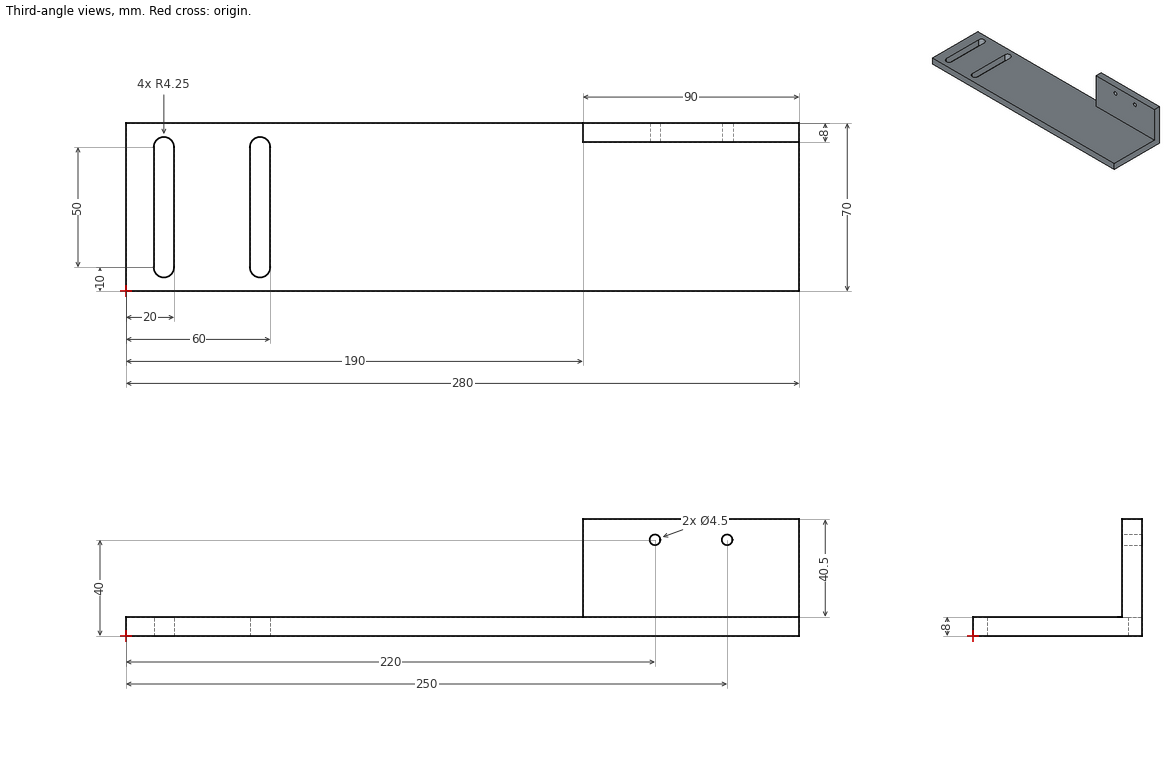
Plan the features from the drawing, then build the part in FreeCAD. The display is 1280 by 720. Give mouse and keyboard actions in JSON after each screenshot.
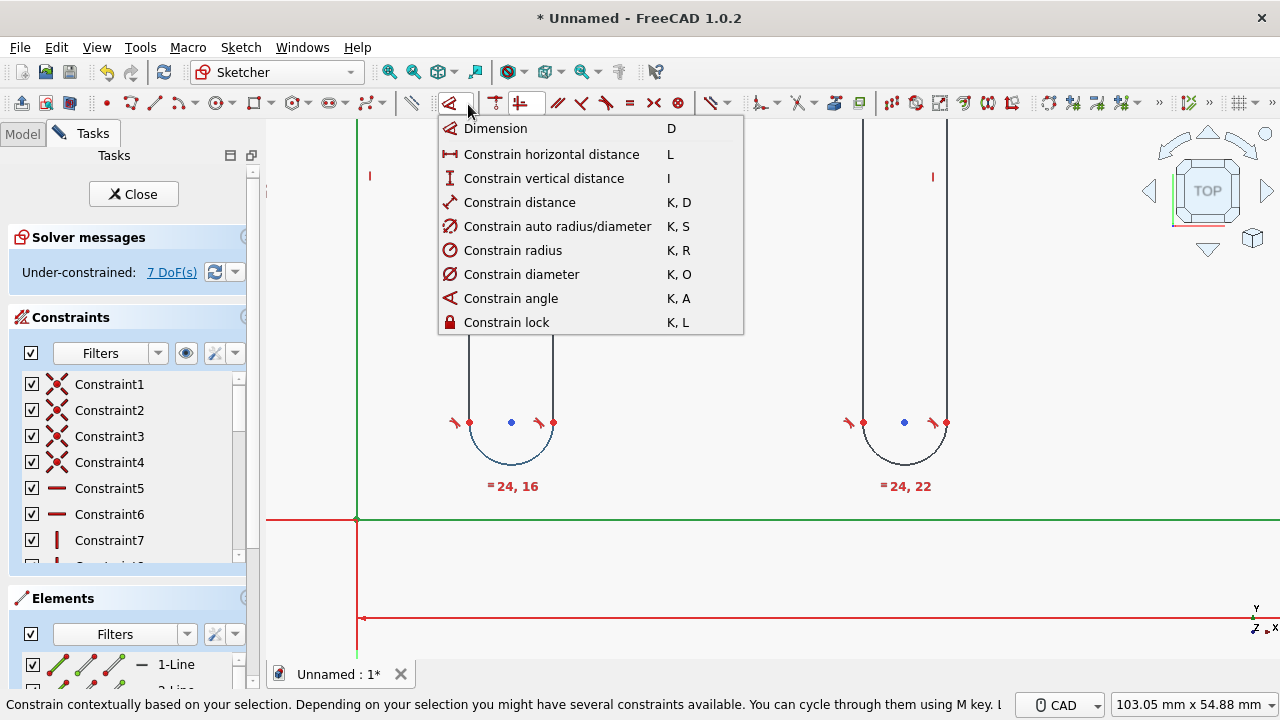
{"action": "left_click", "coordinate": [591, 250]}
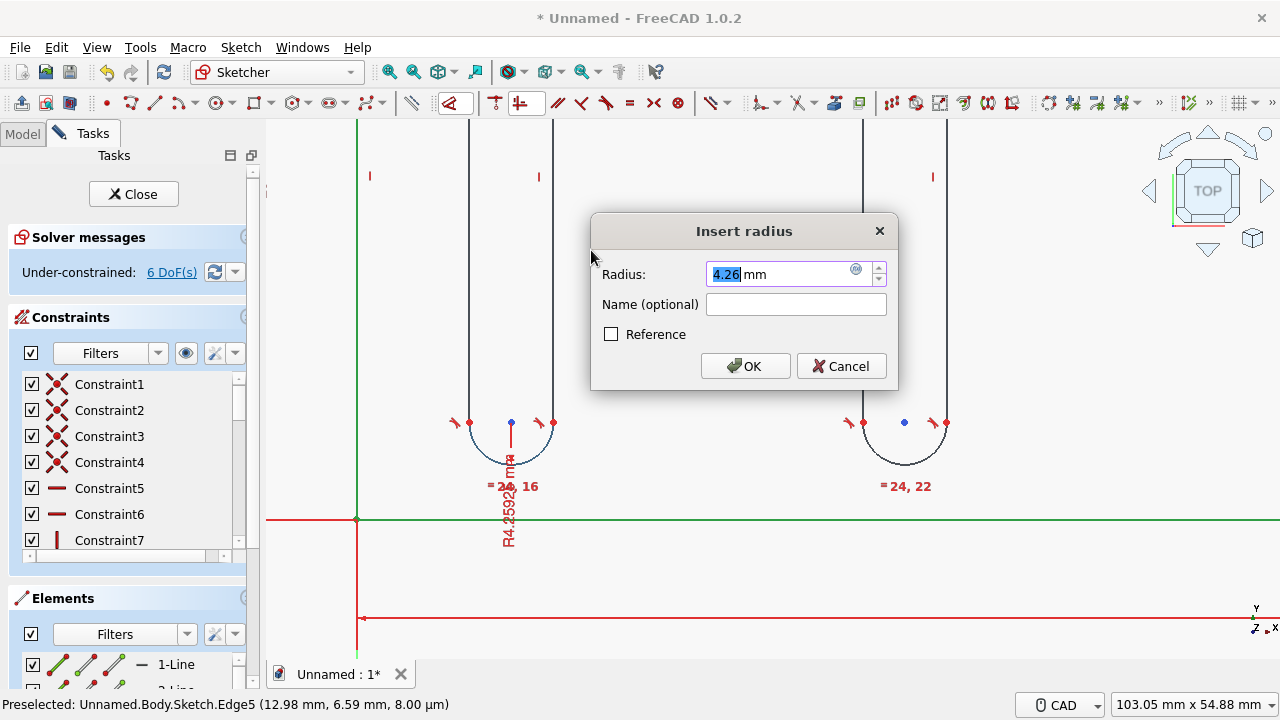
{"action": "type", "text": "4.25"}
{"action": "key", "text": "Return"}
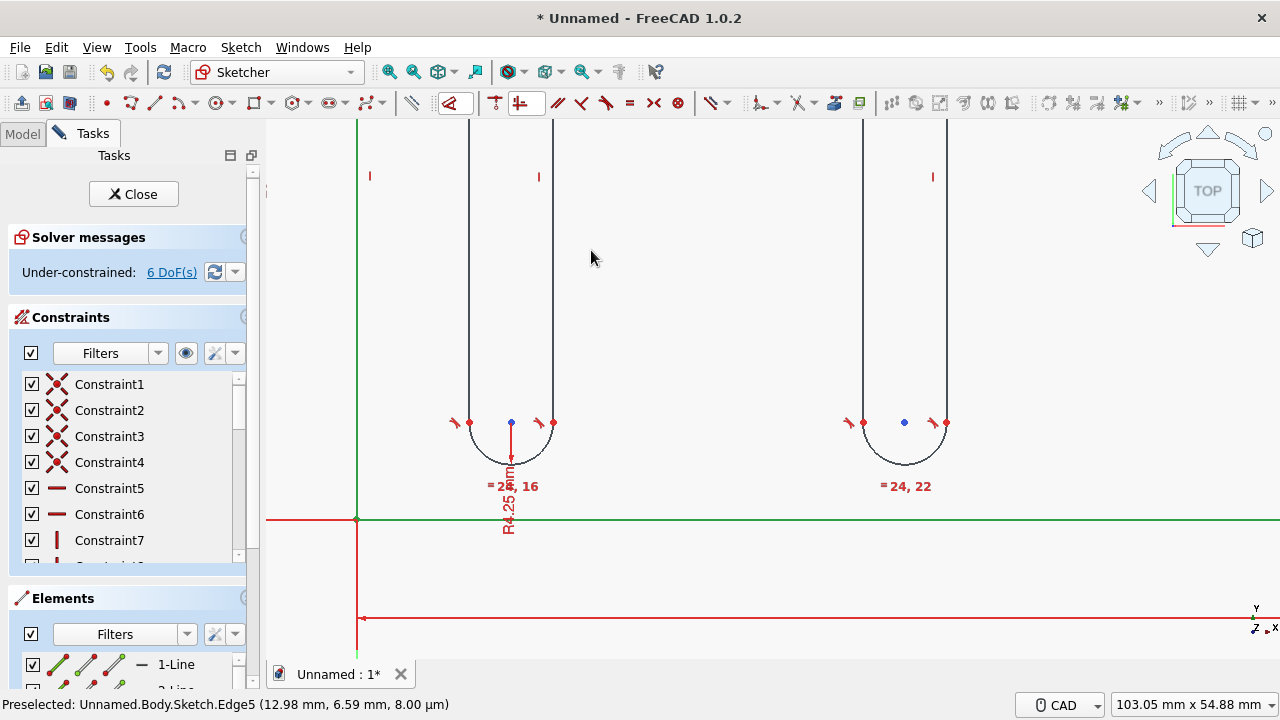
{"action": "scroll", "coordinate": [444, 443], "scroll_direction": "down", "scroll_amount": 8}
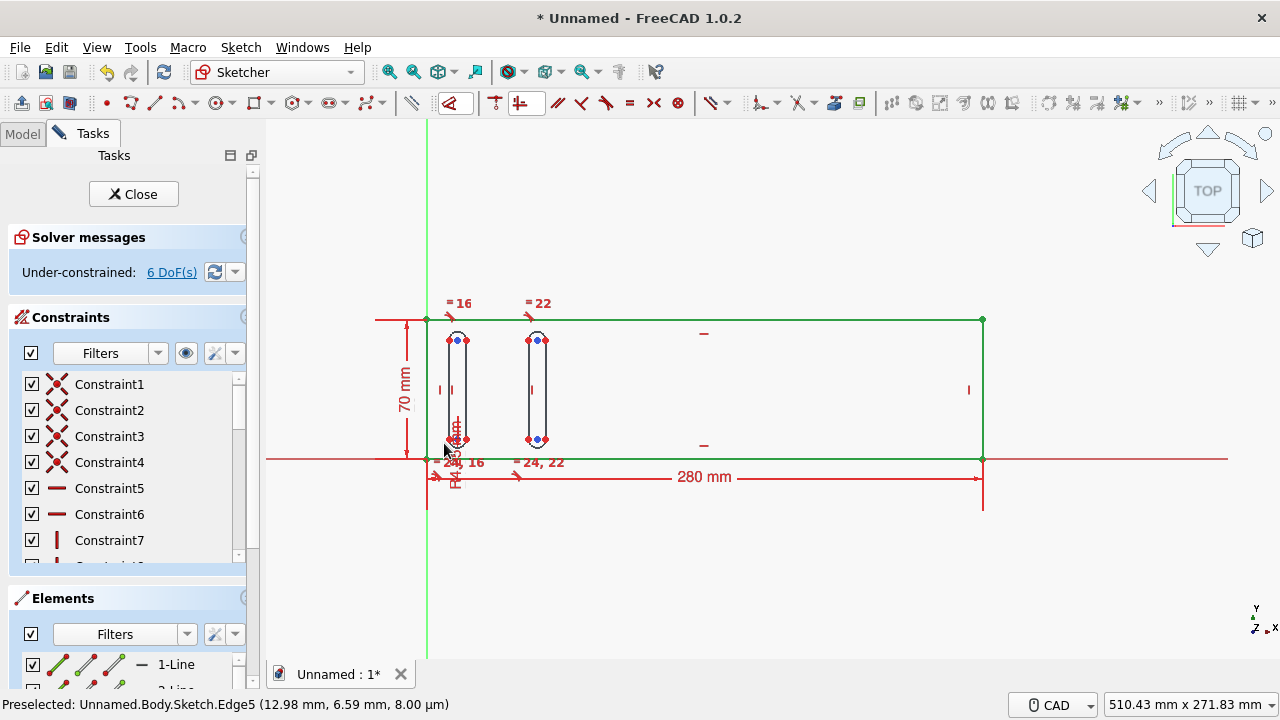
{"action": "left_click", "coordinate": [449, 410]}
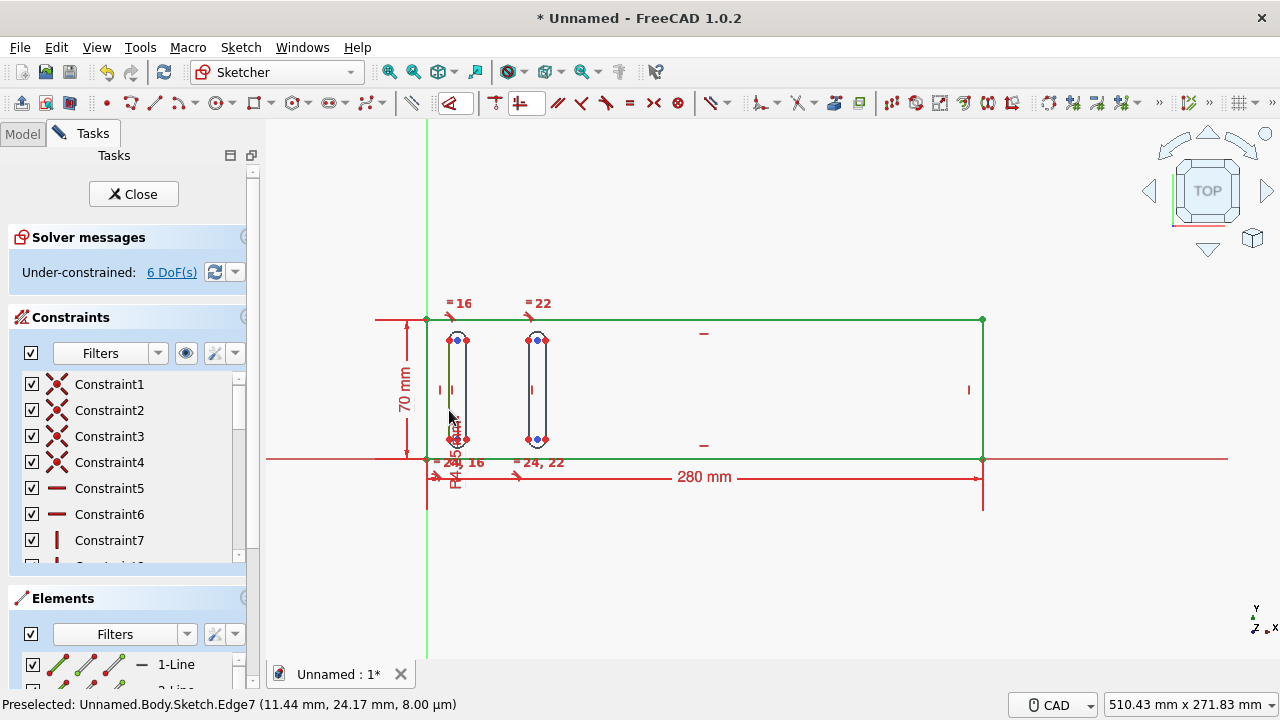
{"action": "key", "text": "i"}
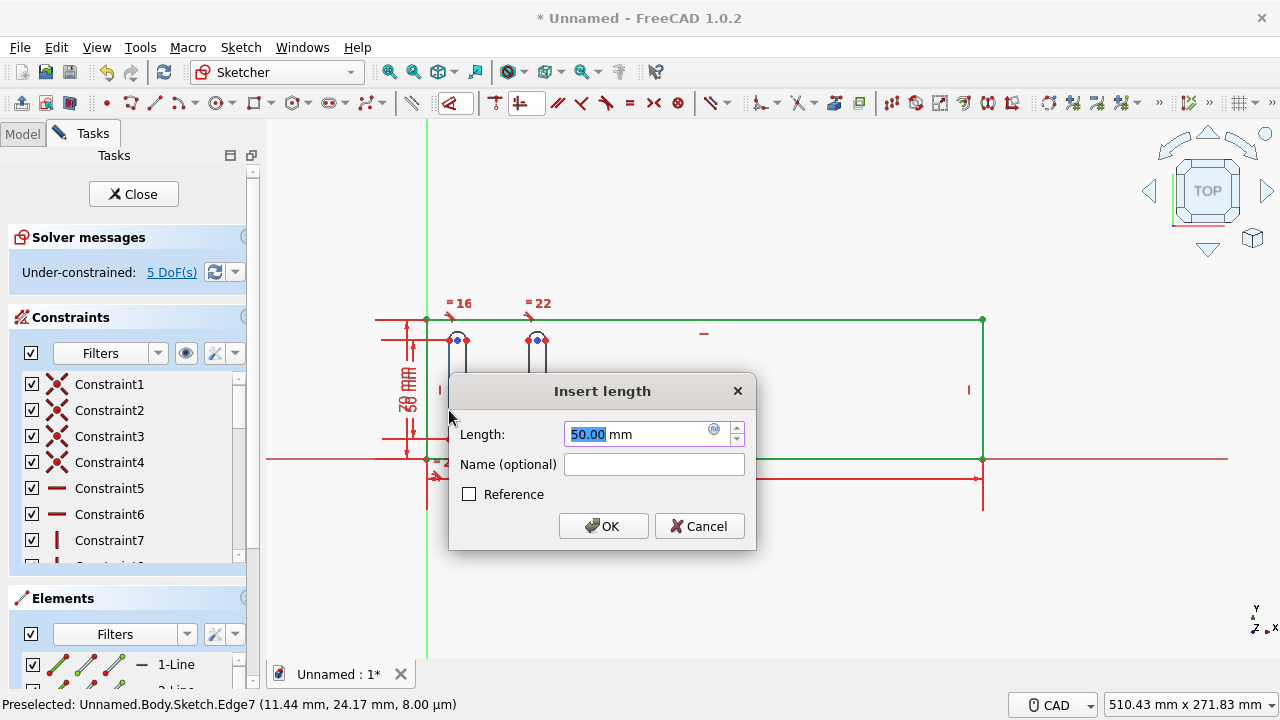
{"action": "type", "text": "50"}
{"action": "key", "text": "Return"}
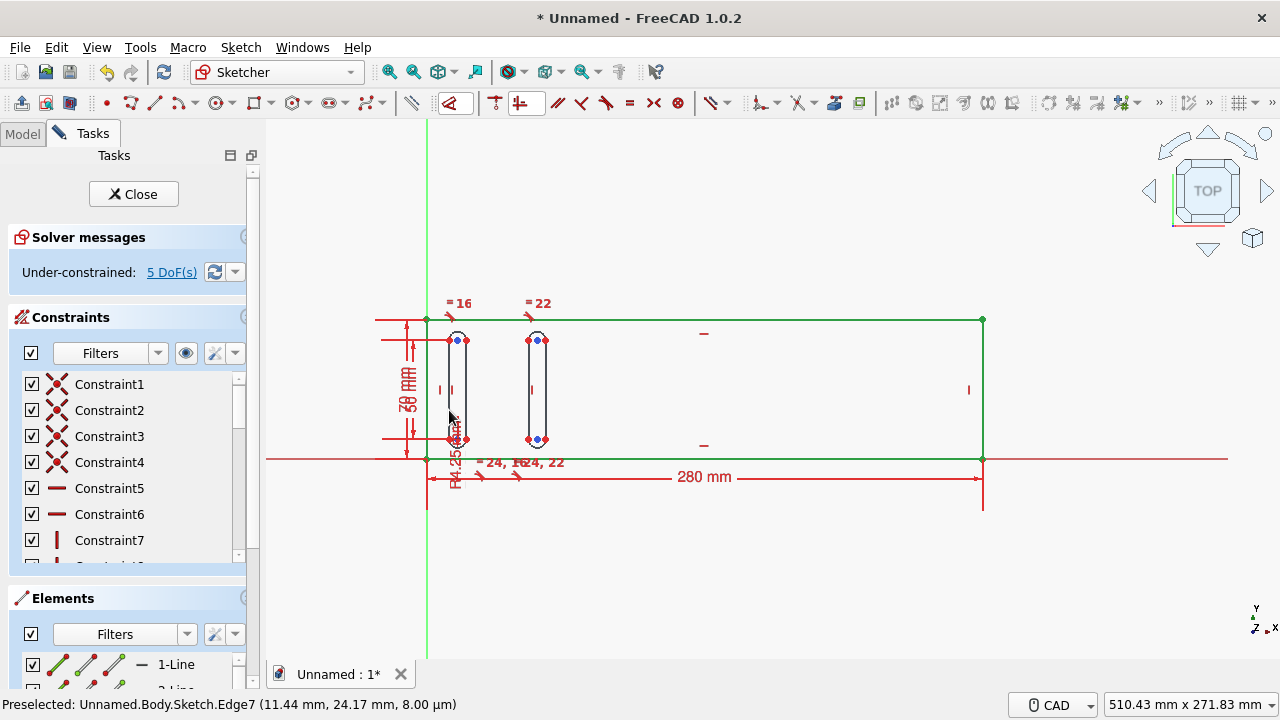
{"action": "left_click", "coordinate": [529, 410]}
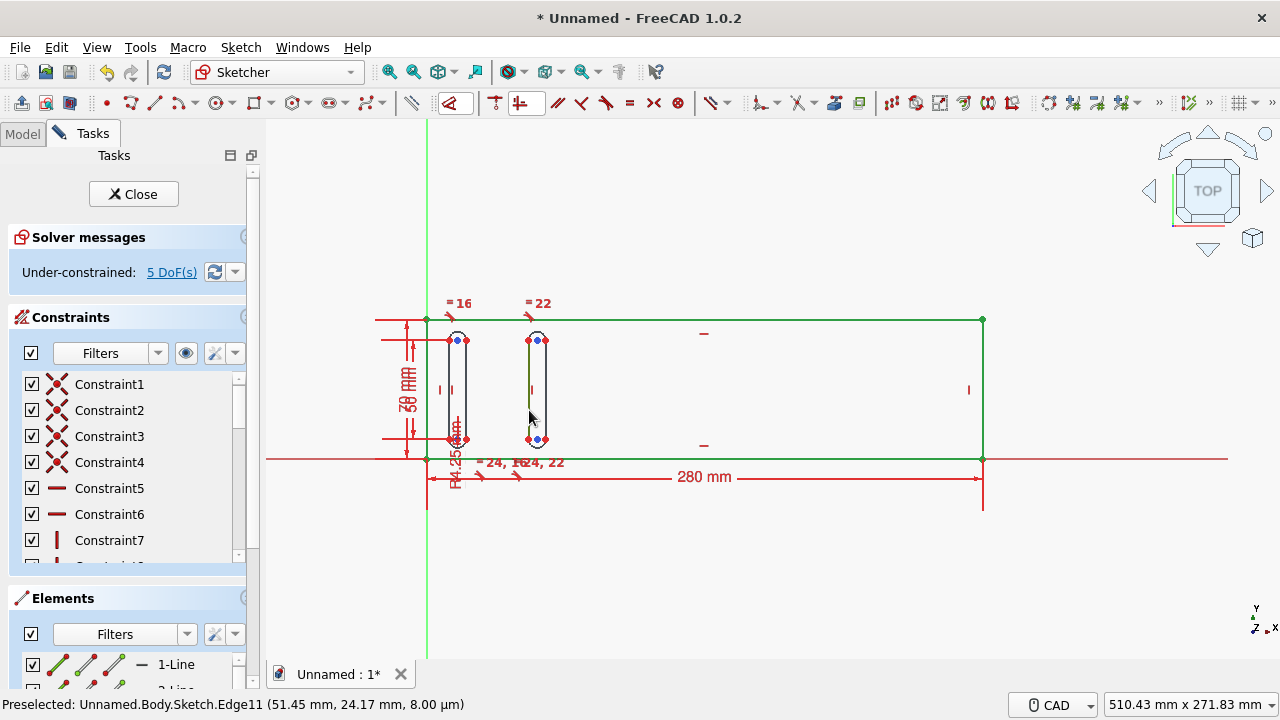
{"action": "key", "text": "i"}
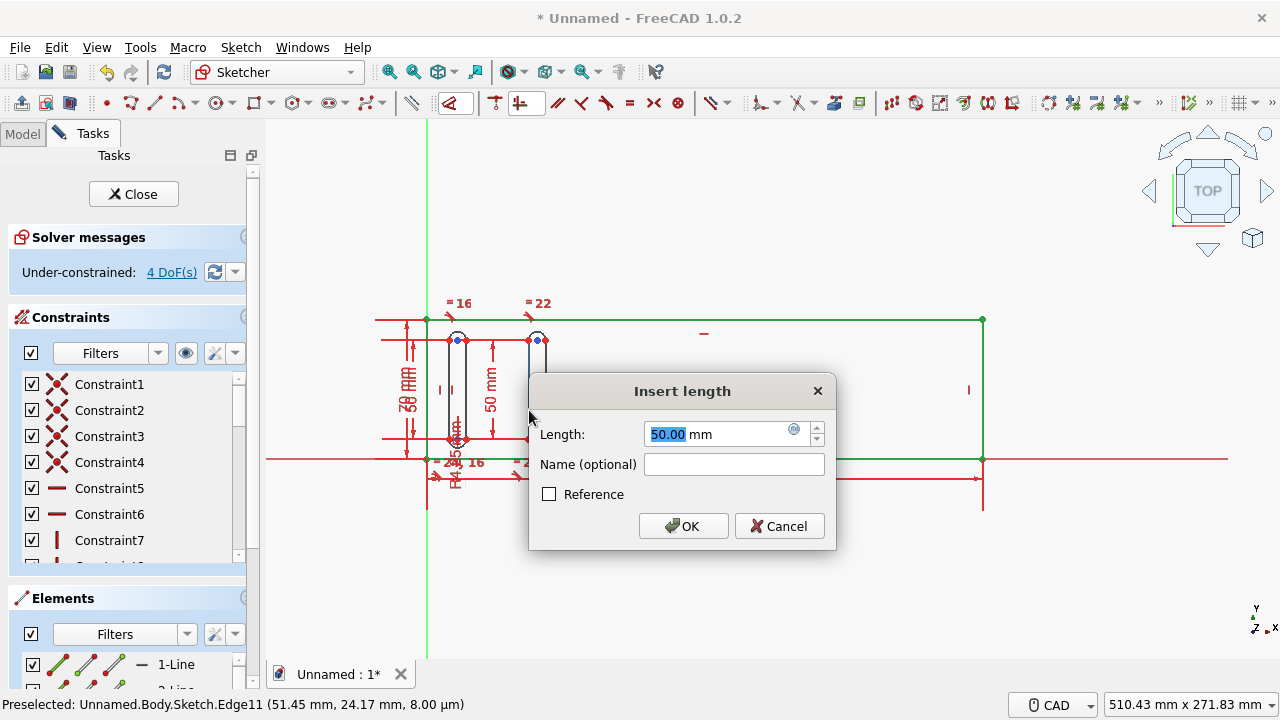
{"action": "type", "text": "50"}
{"action": "key", "text": "Return"}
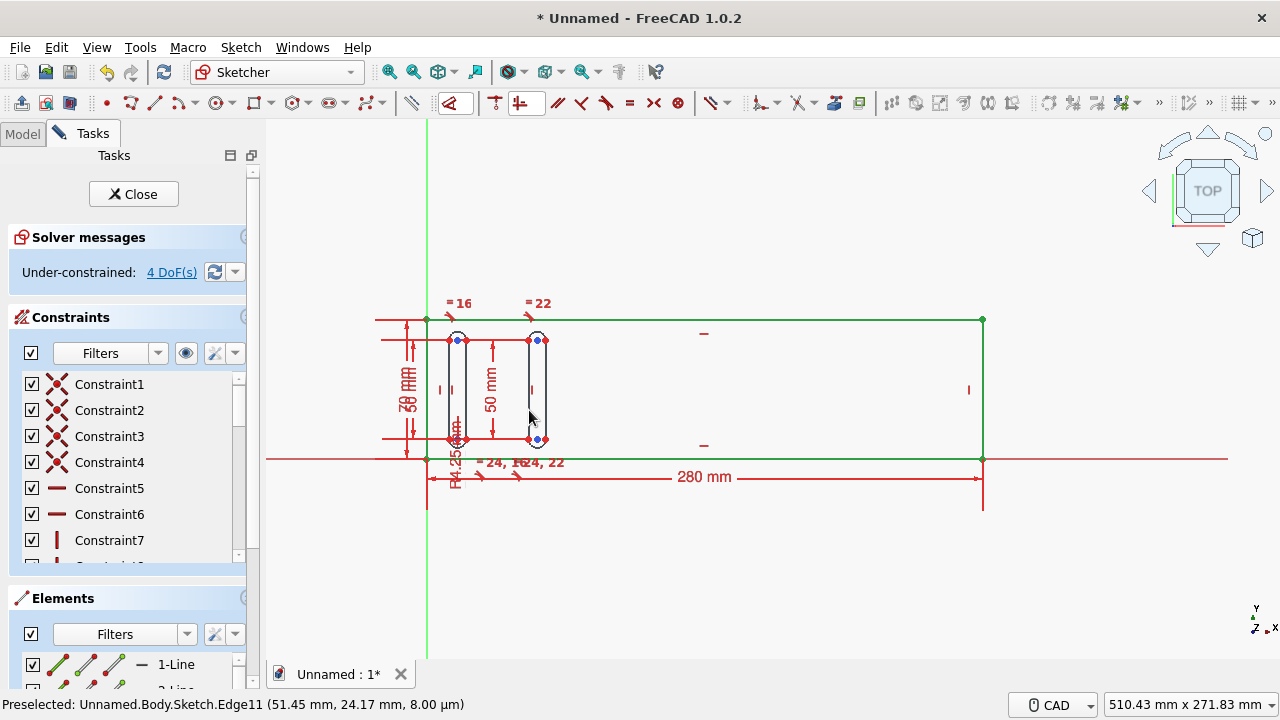
{"action": "scroll", "coordinate": [449, 439], "scroll_direction": "up", "scroll_amount": 4}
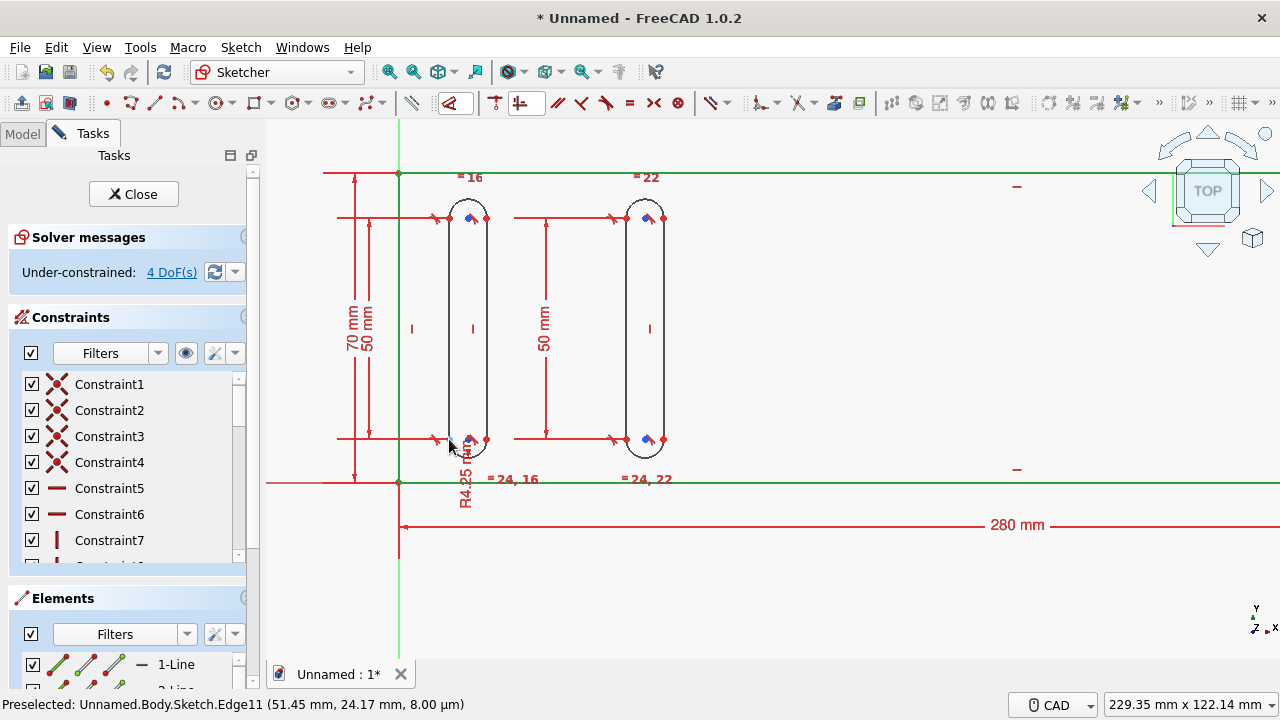
{"action": "left_click", "coordinate": [449, 439]}